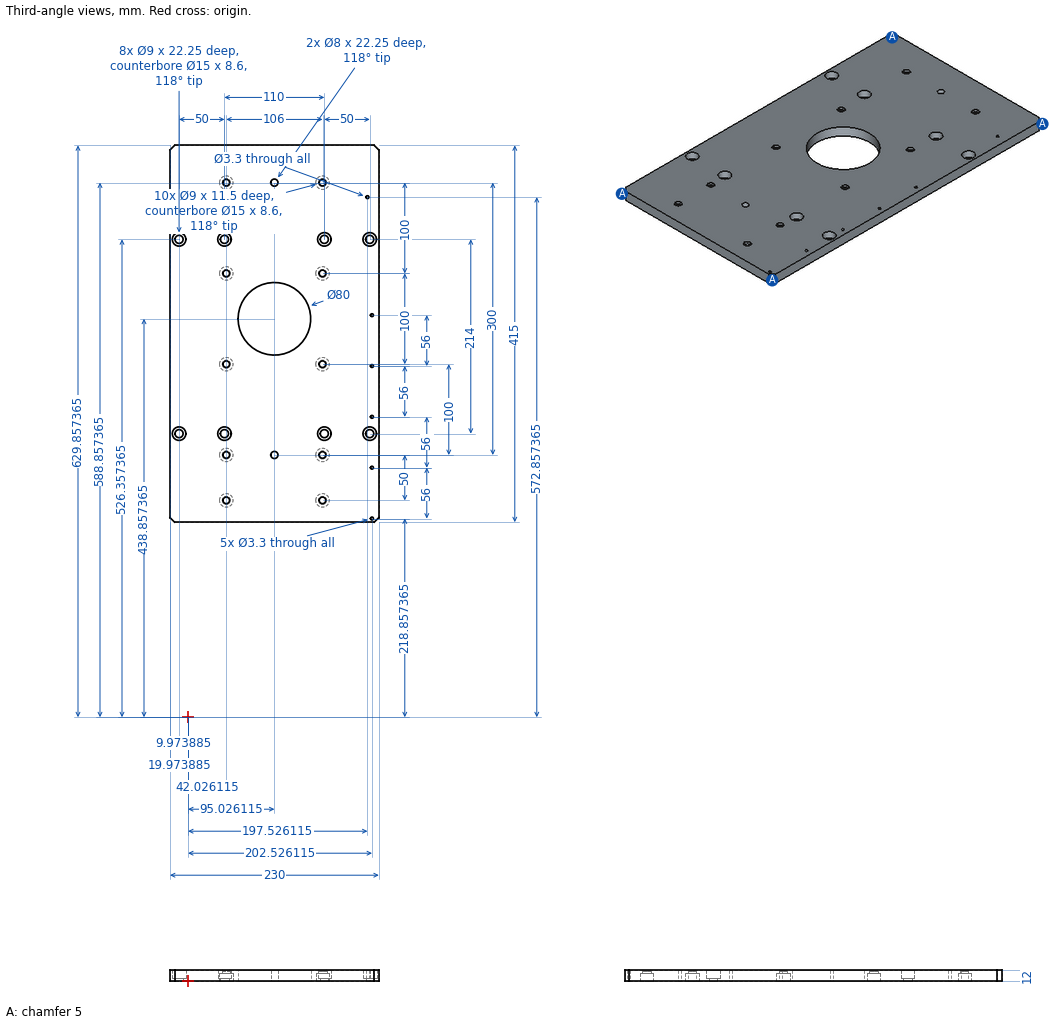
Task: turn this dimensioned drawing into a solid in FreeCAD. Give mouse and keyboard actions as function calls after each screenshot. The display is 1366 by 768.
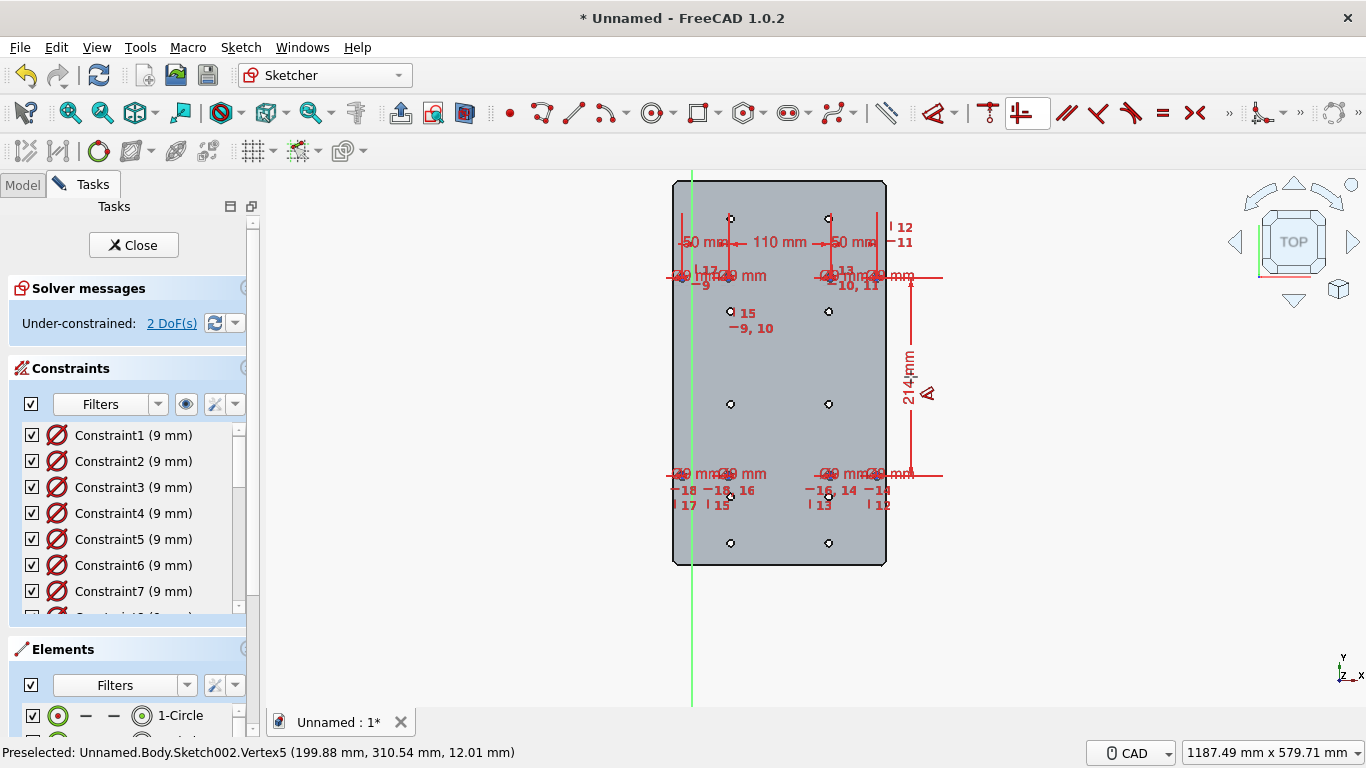
scroll(682, 278, up, 8)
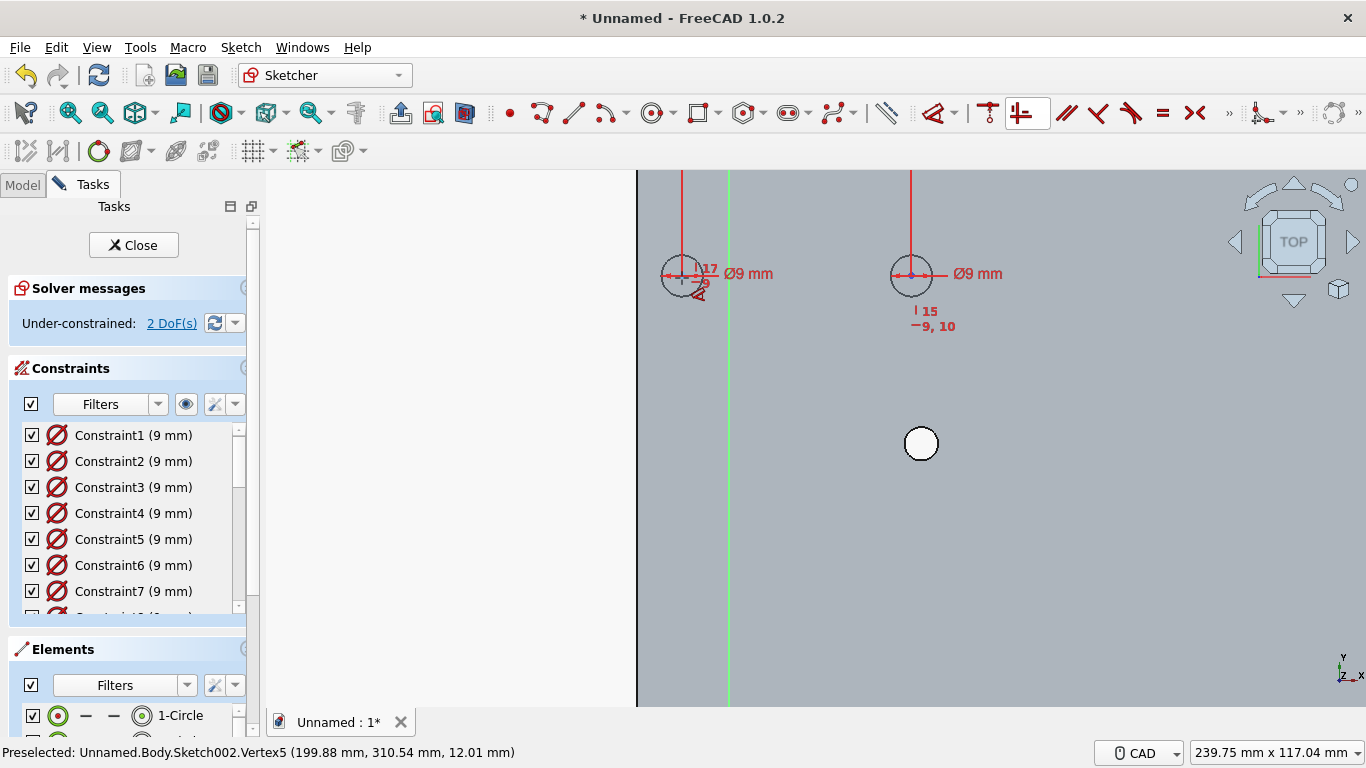
click(682, 276)
click(705, 242)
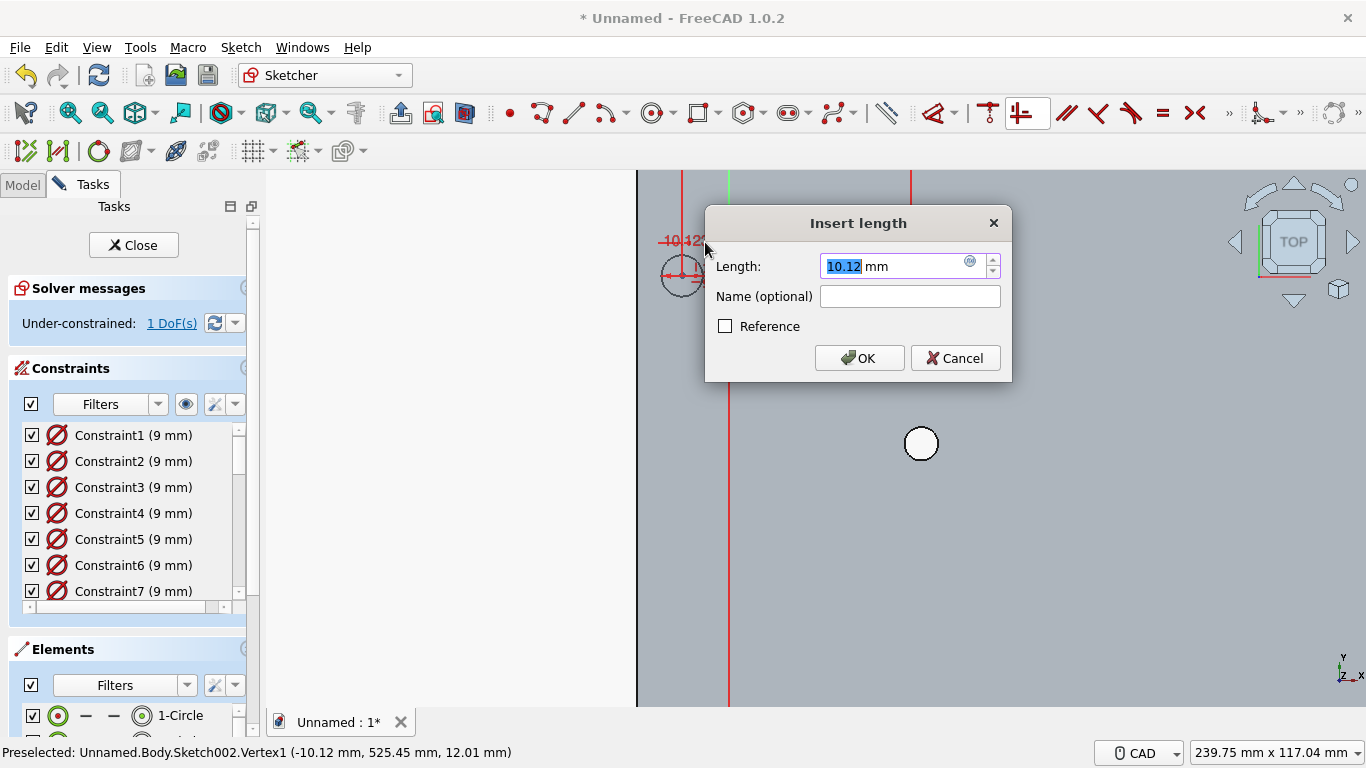
text(9.973885)
key(Return)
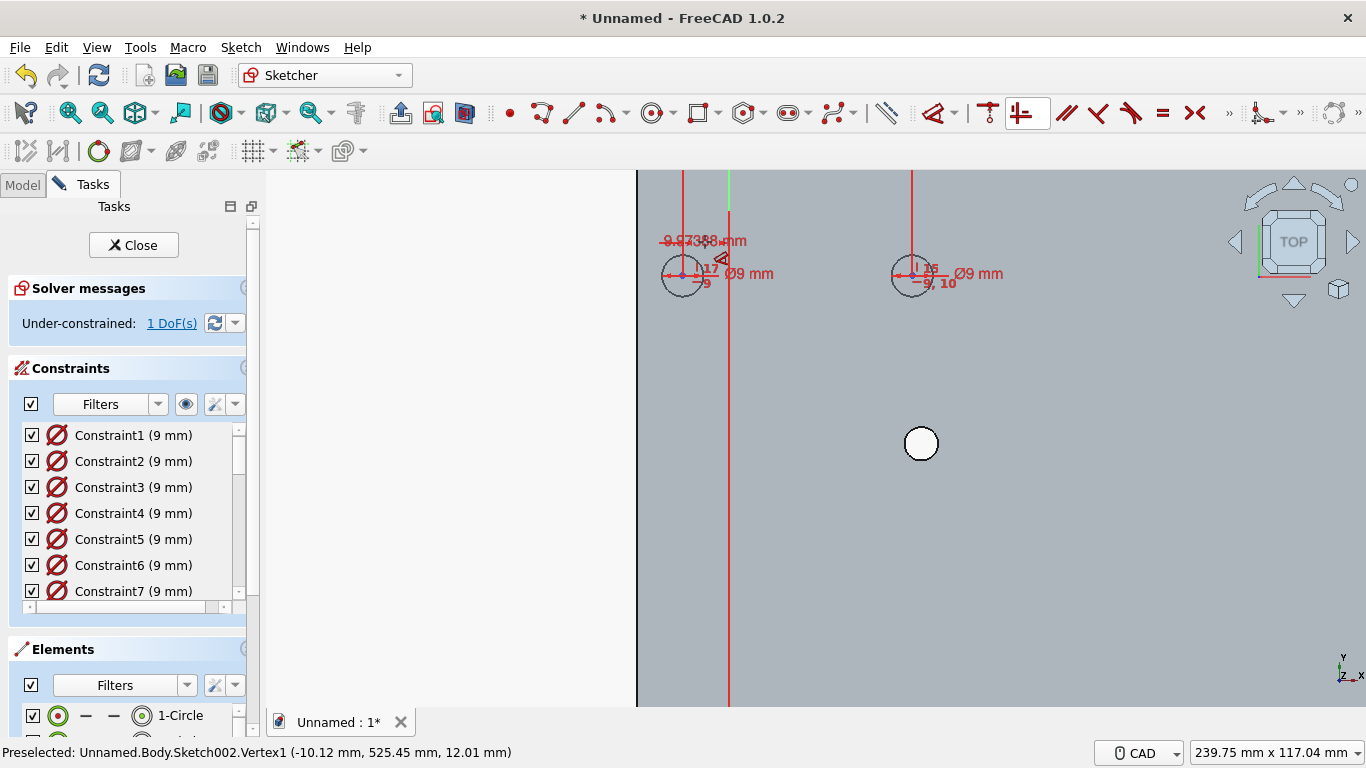
scroll(682, 277, down, 10)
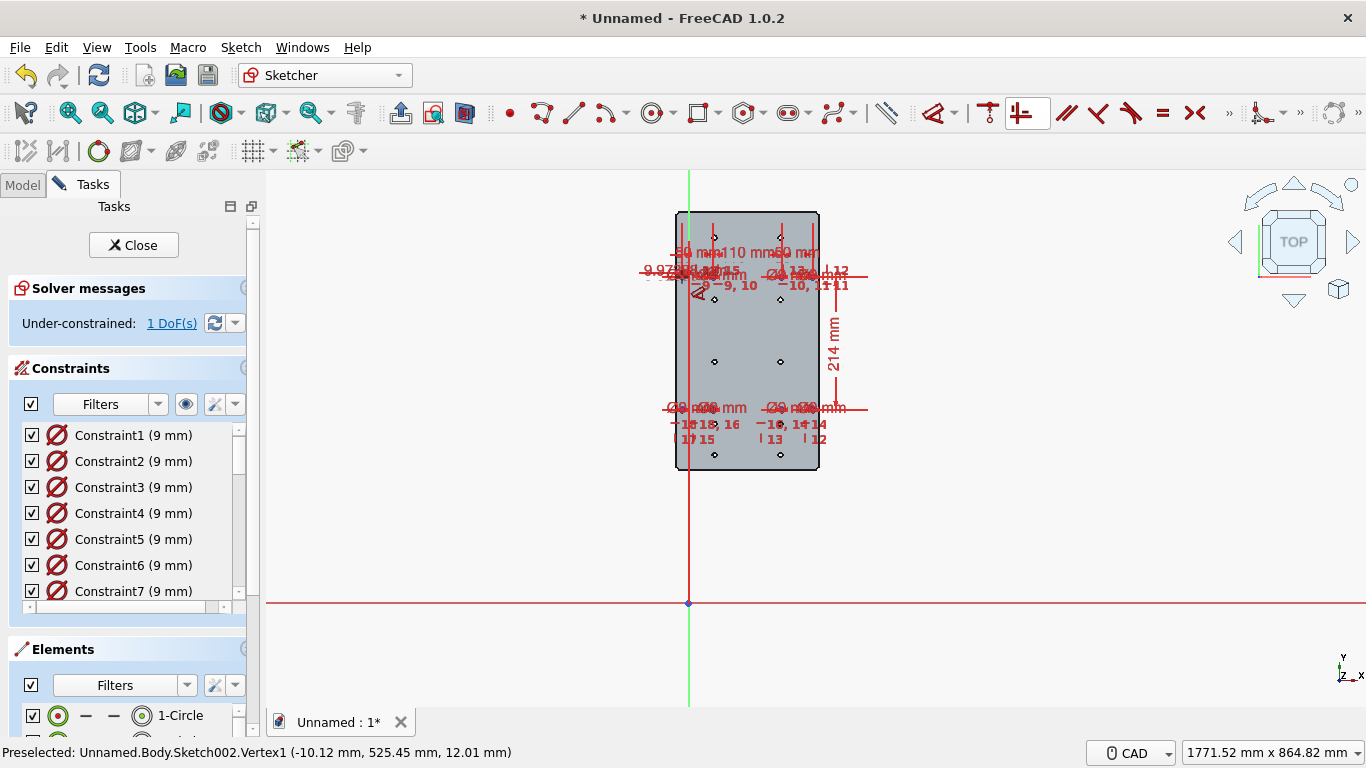
click(682, 277)
click(648, 440)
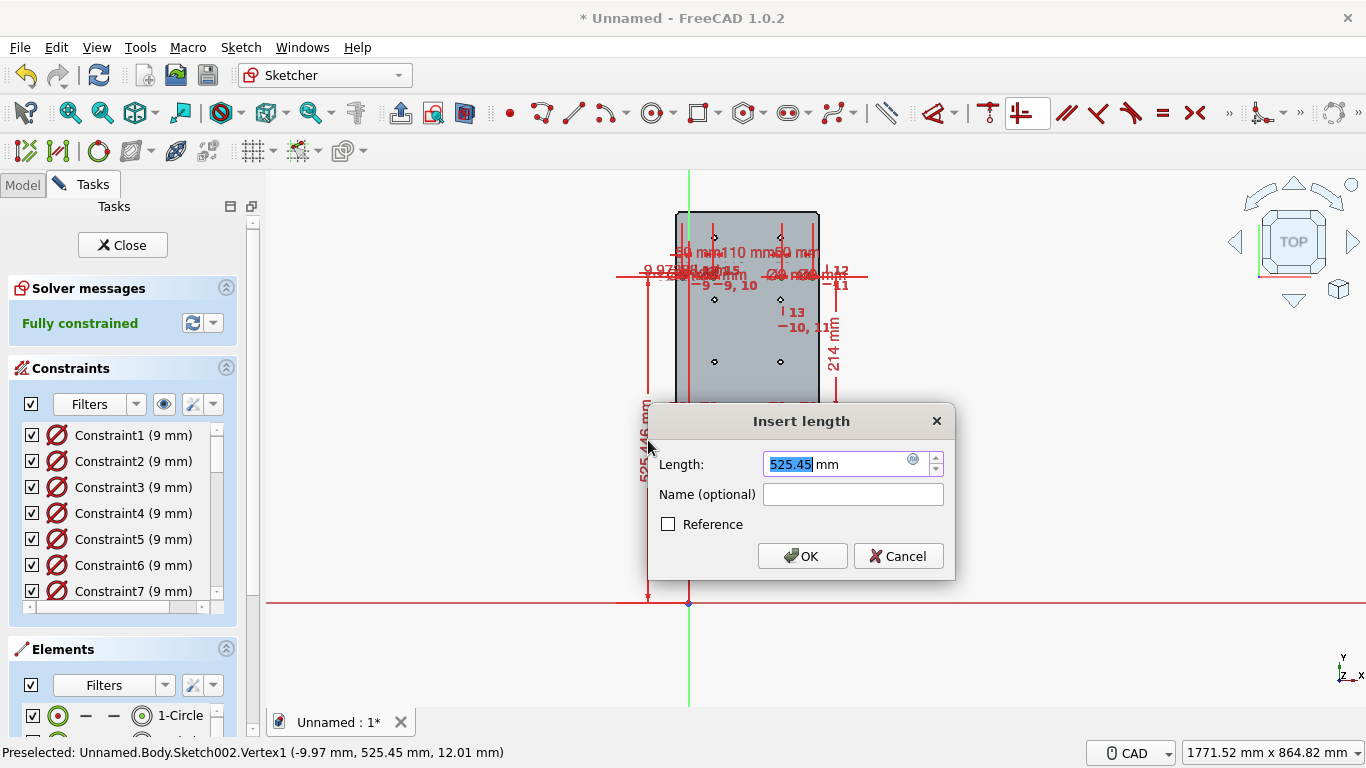
text(526.357365)
key(Return)
key(Escape)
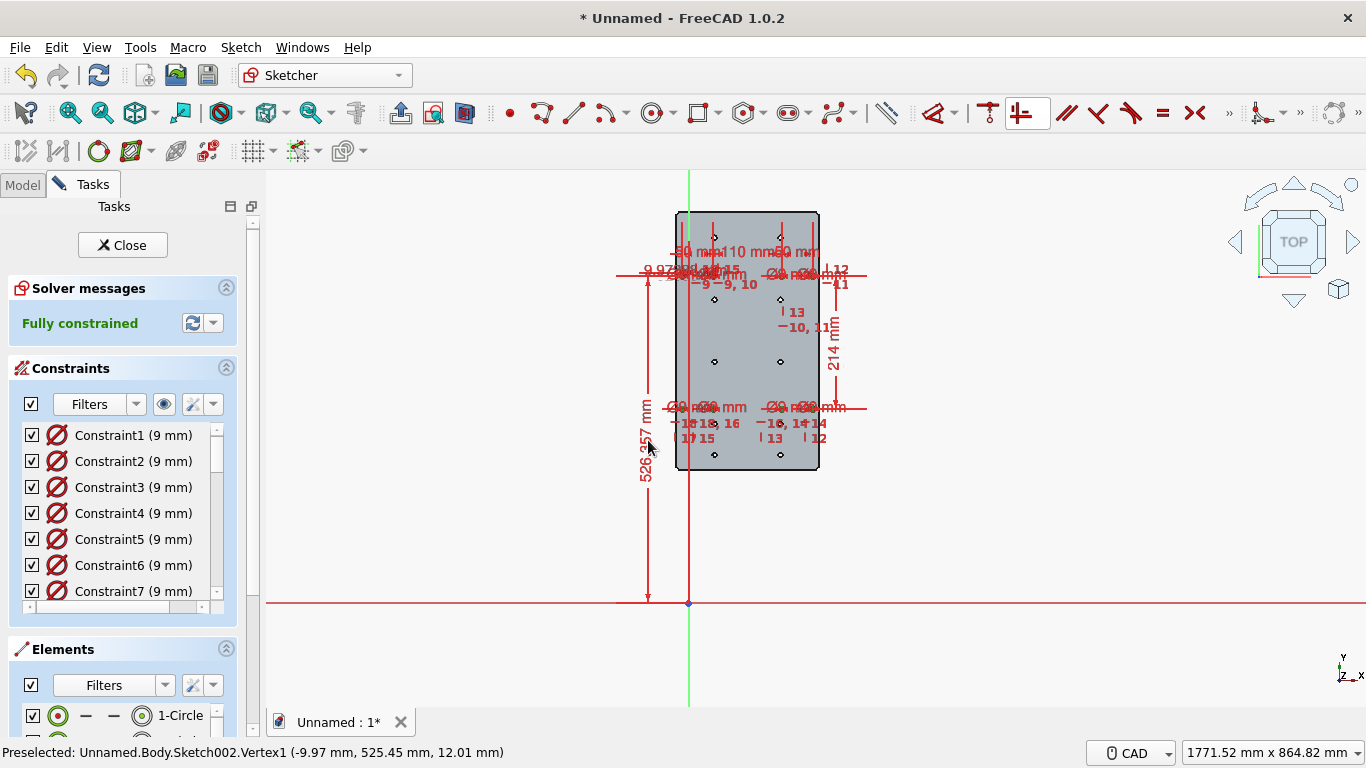
click(123, 245)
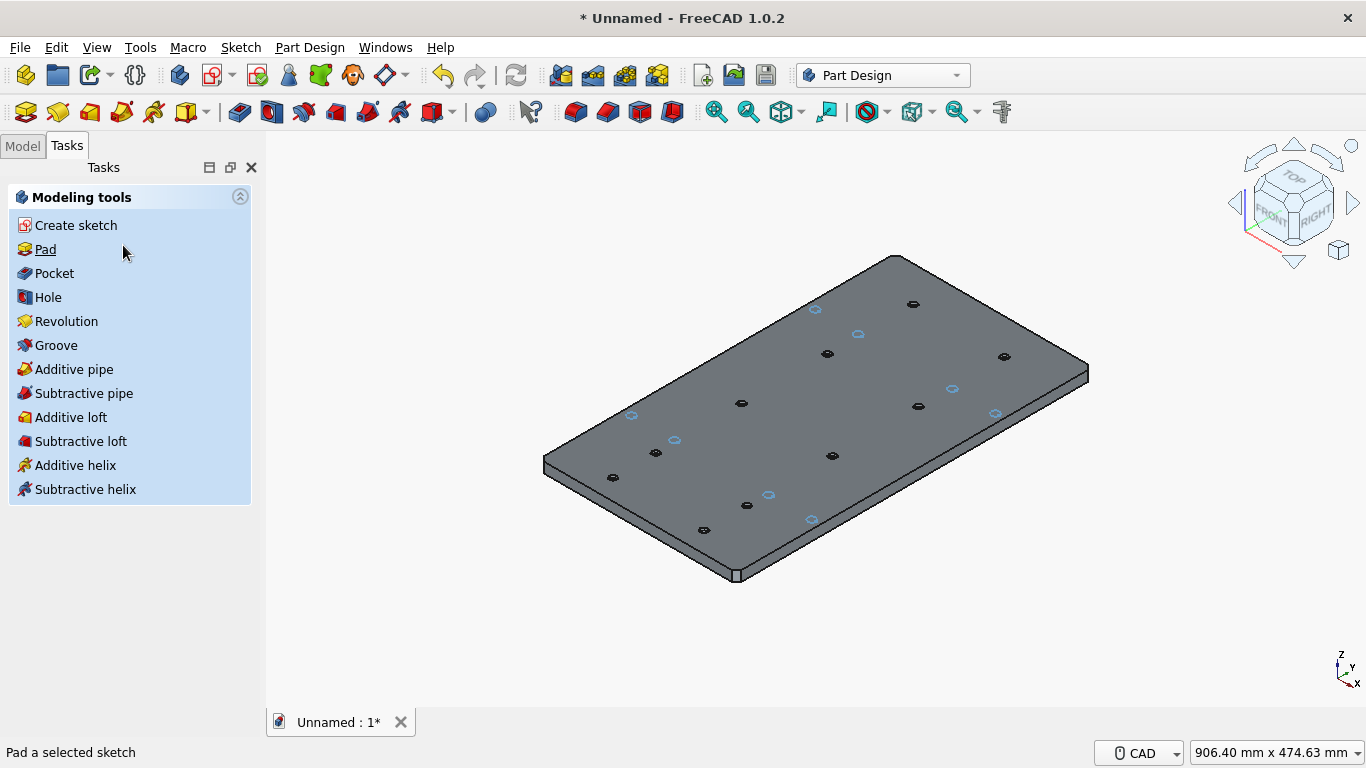
click(272, 112)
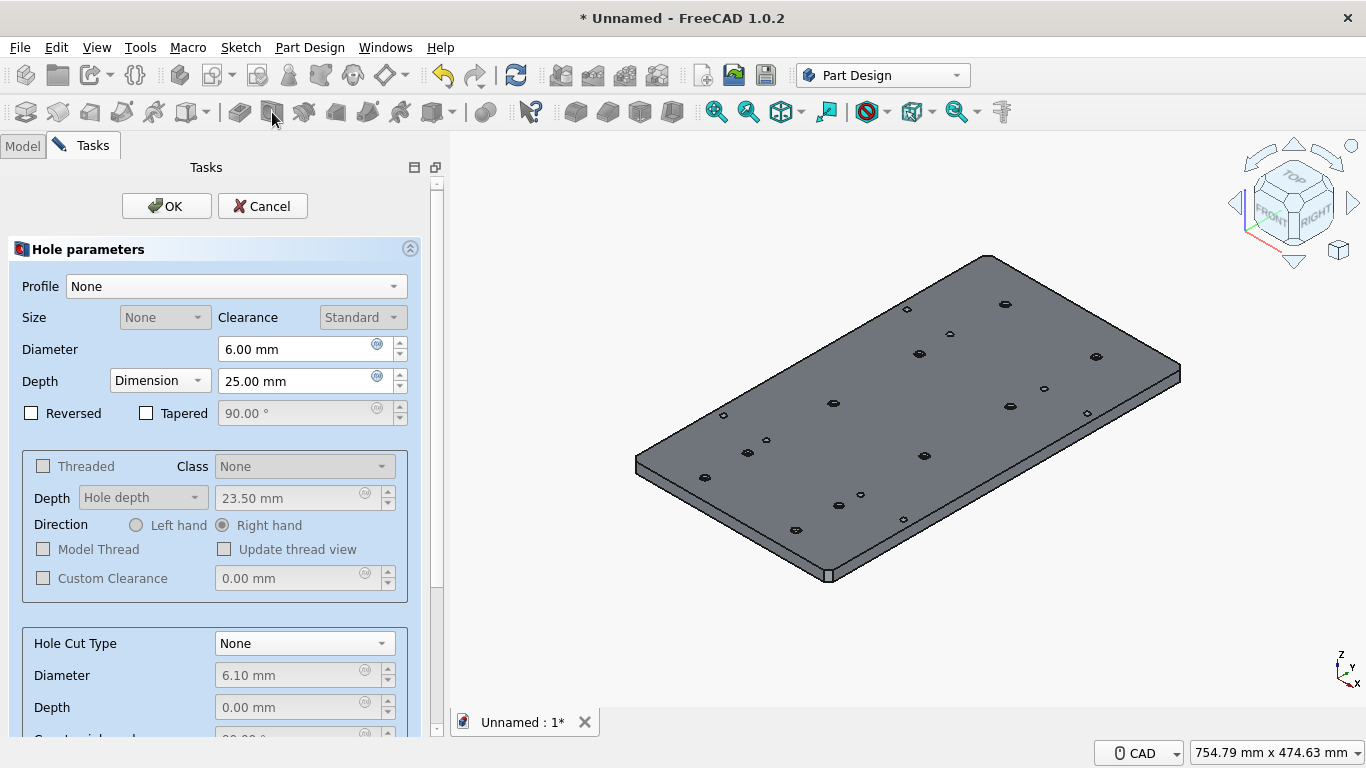
triple_click(305, 349)